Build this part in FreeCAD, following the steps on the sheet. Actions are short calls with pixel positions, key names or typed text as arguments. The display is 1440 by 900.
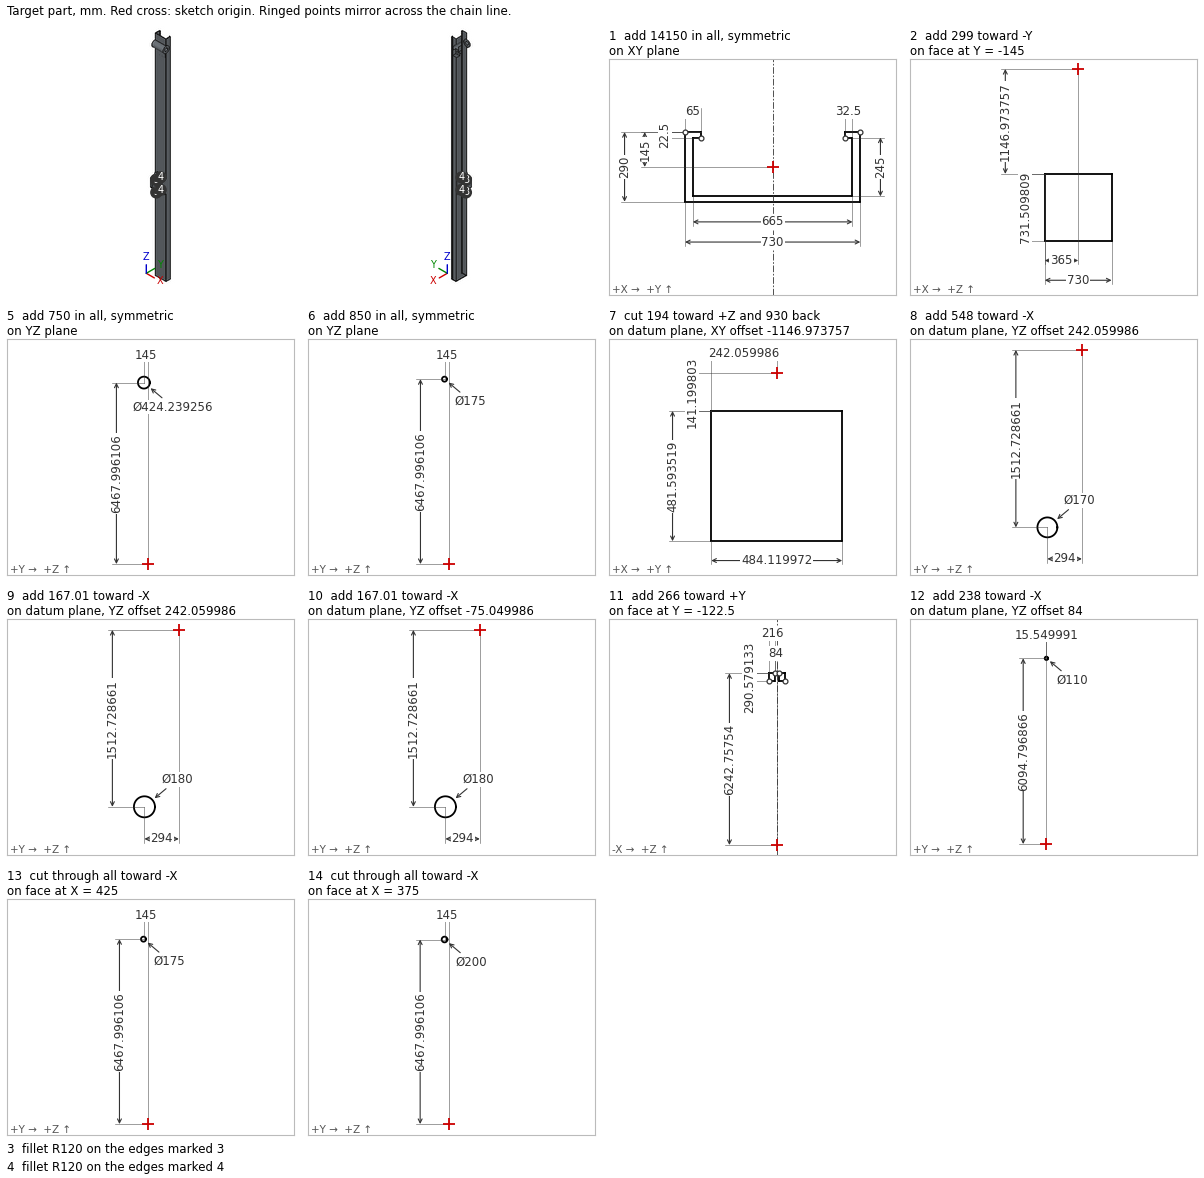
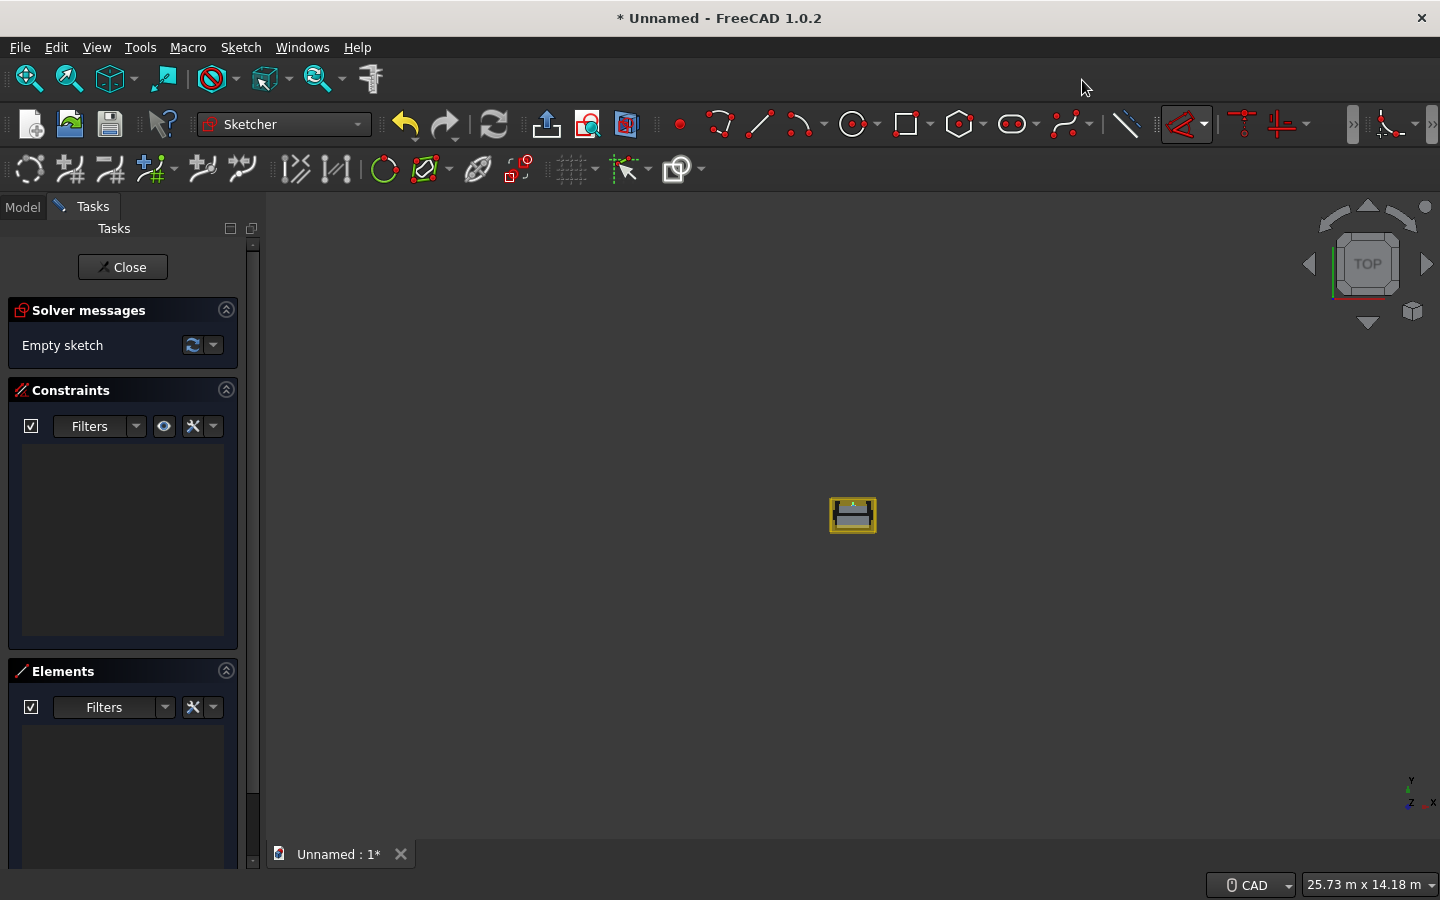
click(628, 124)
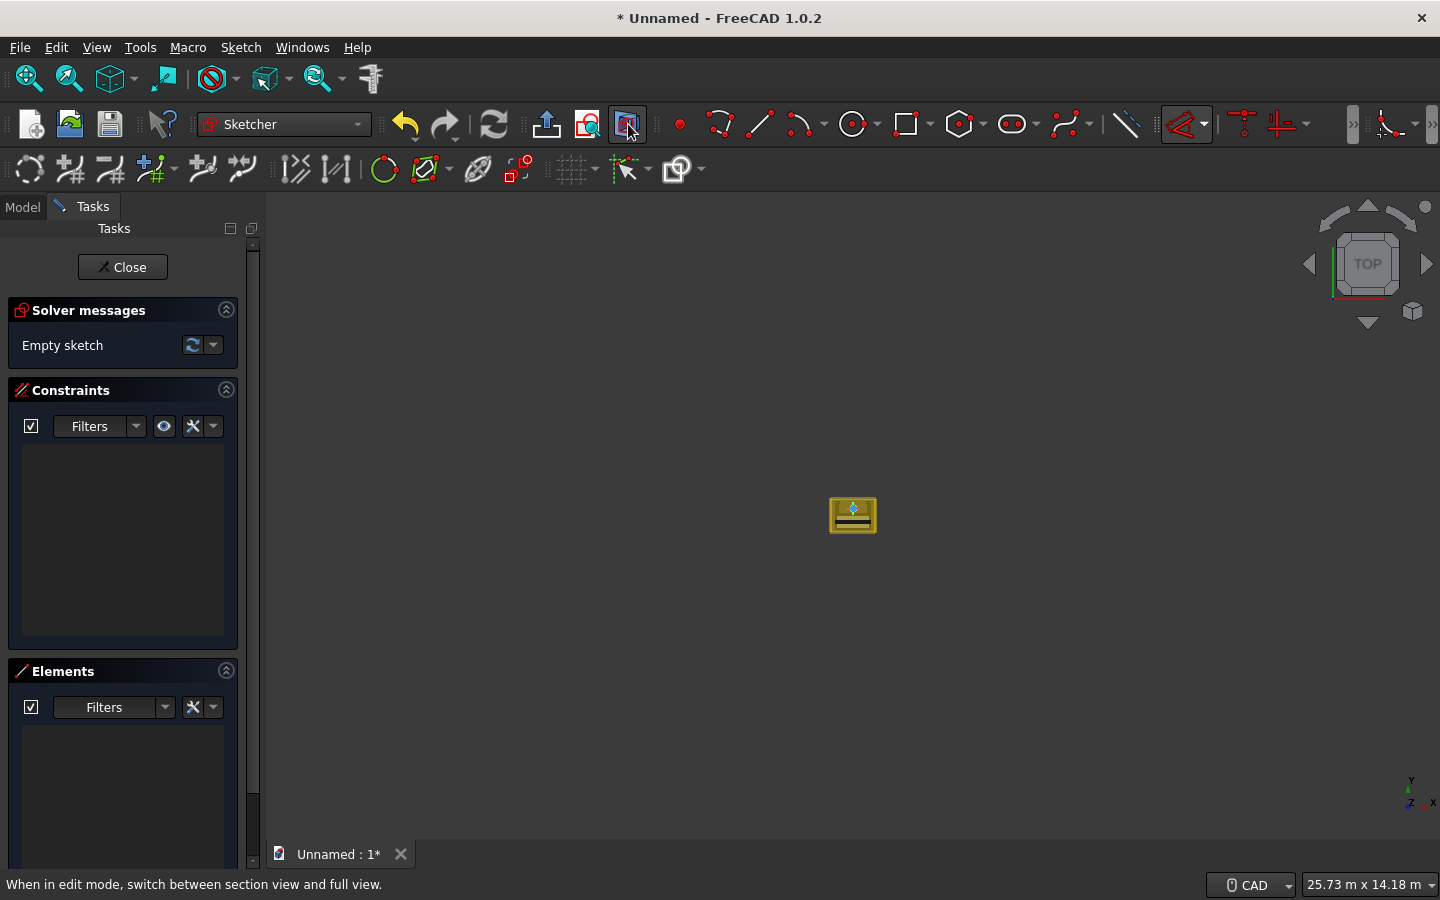
scroll(858, 523, up, 13)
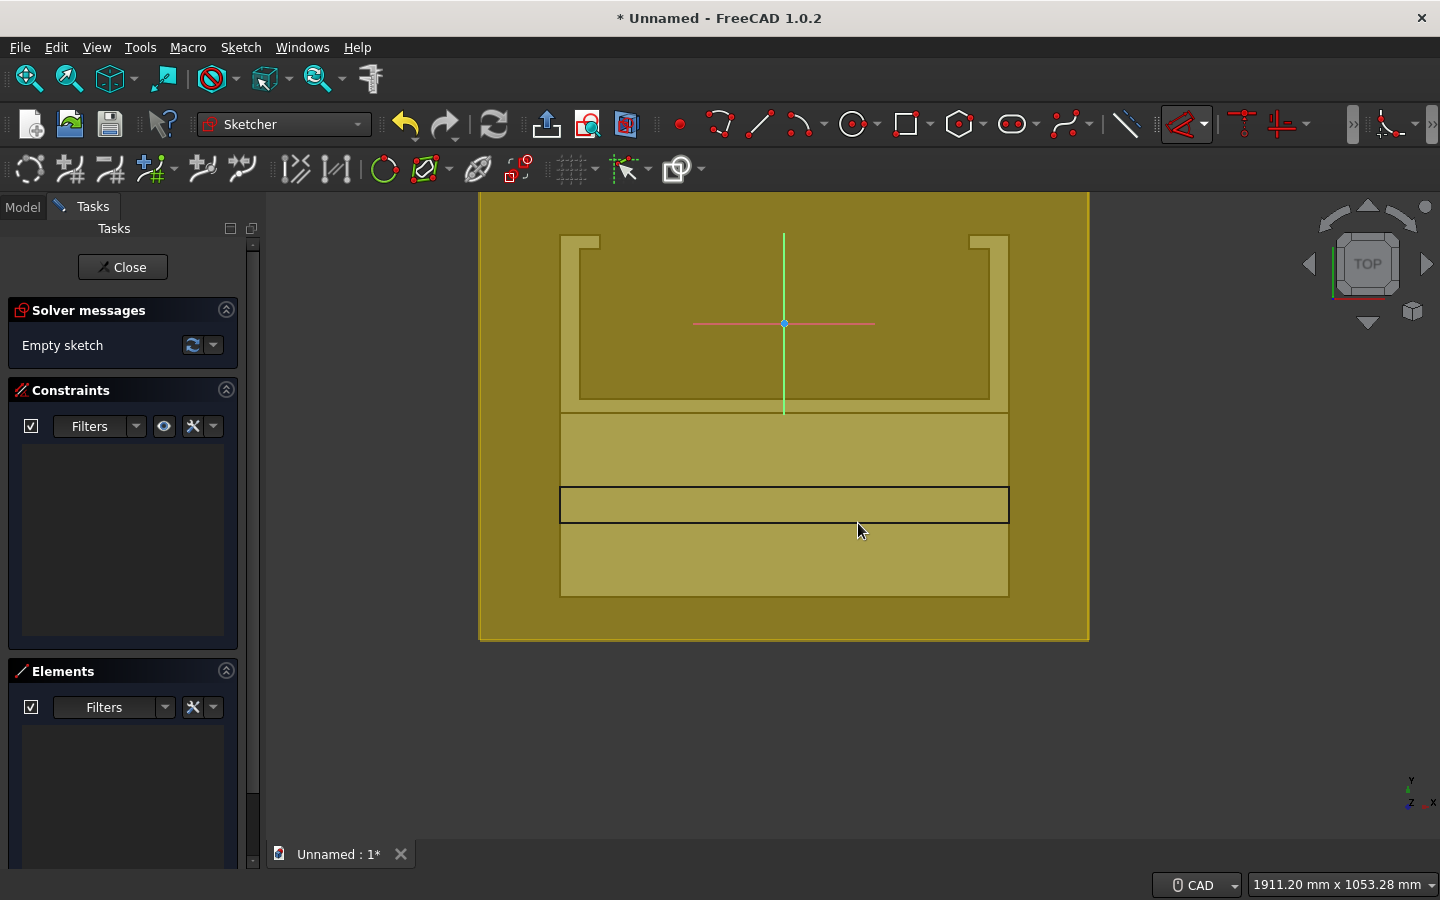
key(g)
key(r)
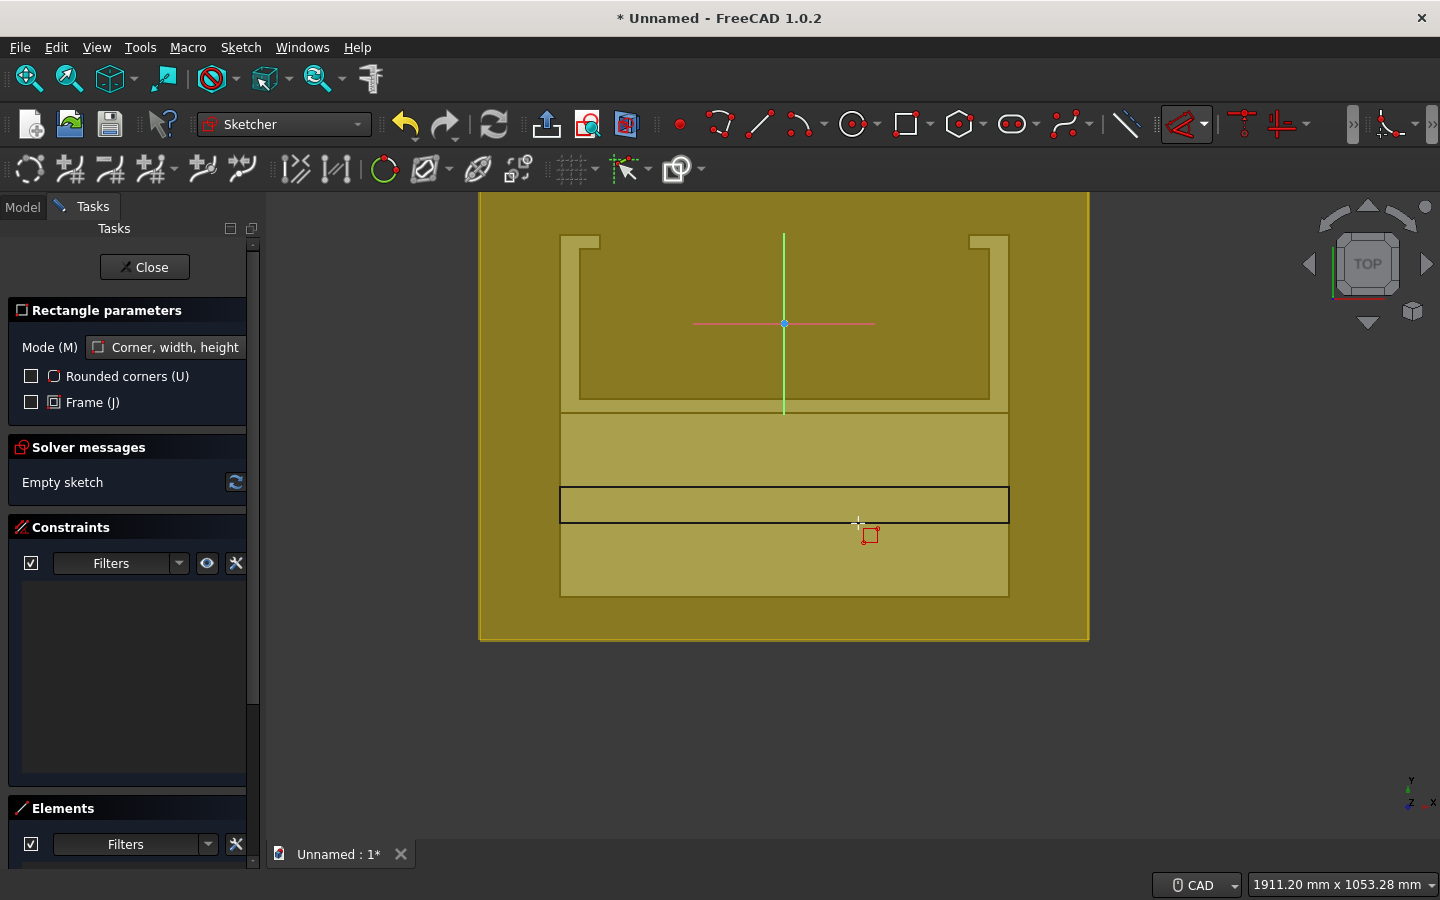
click(636, 411)
click(933, 706)
key(Escape)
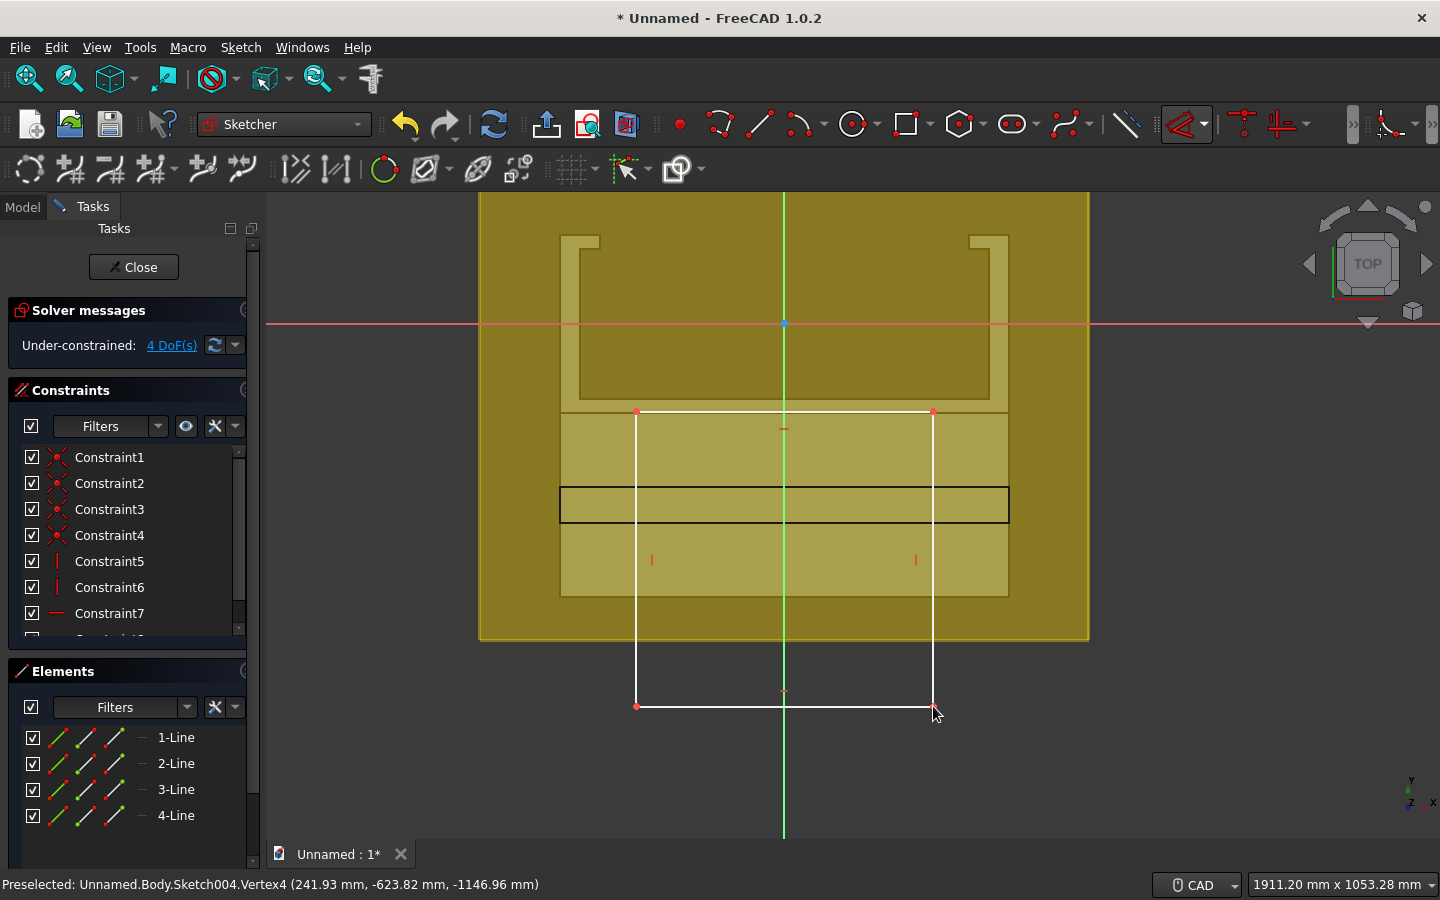
click(636, 500)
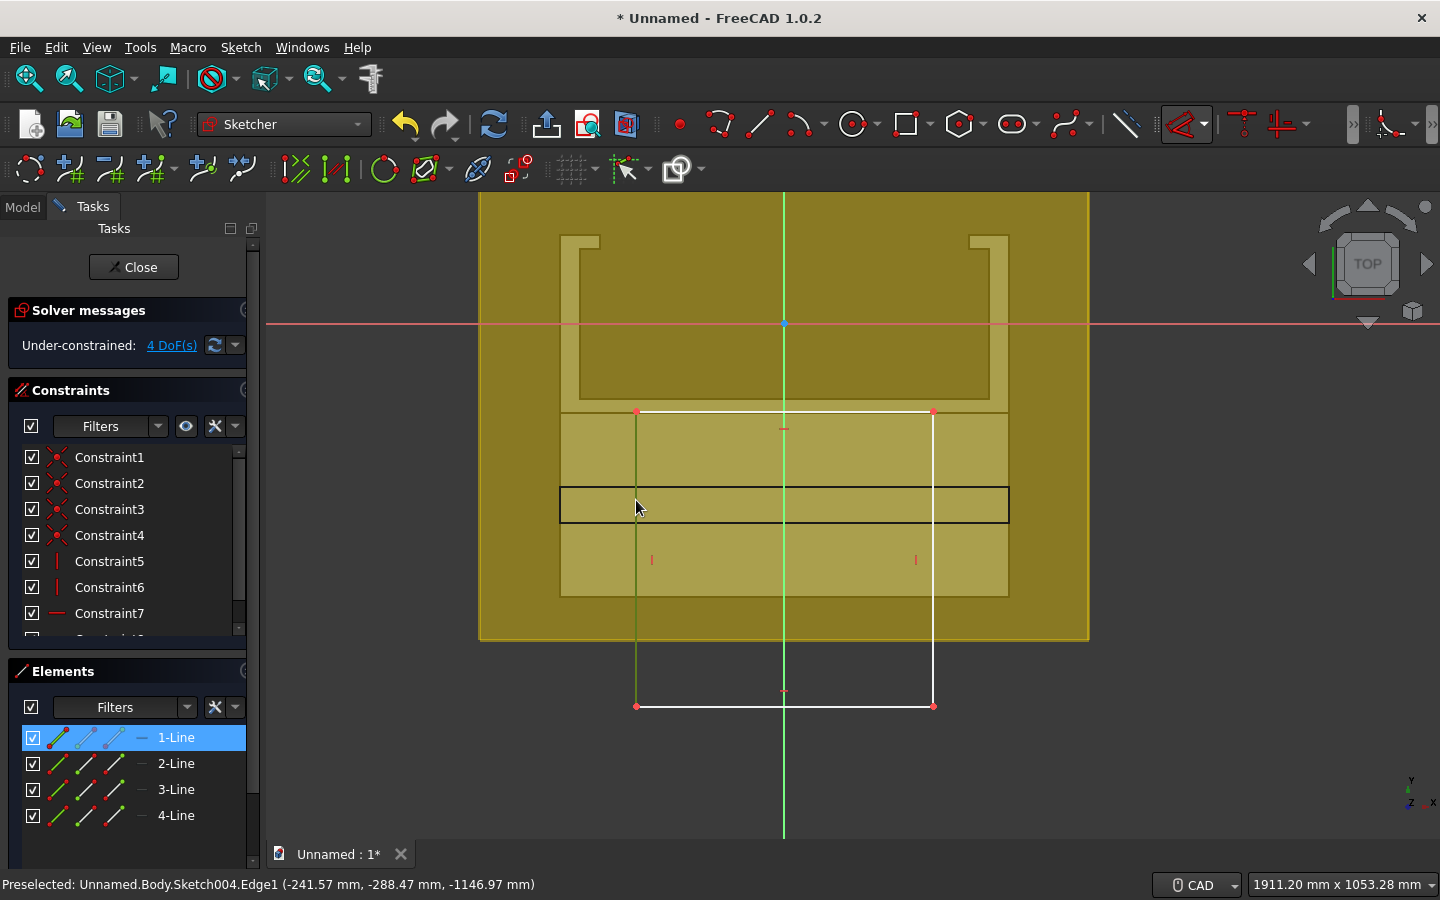
click(1206, 124)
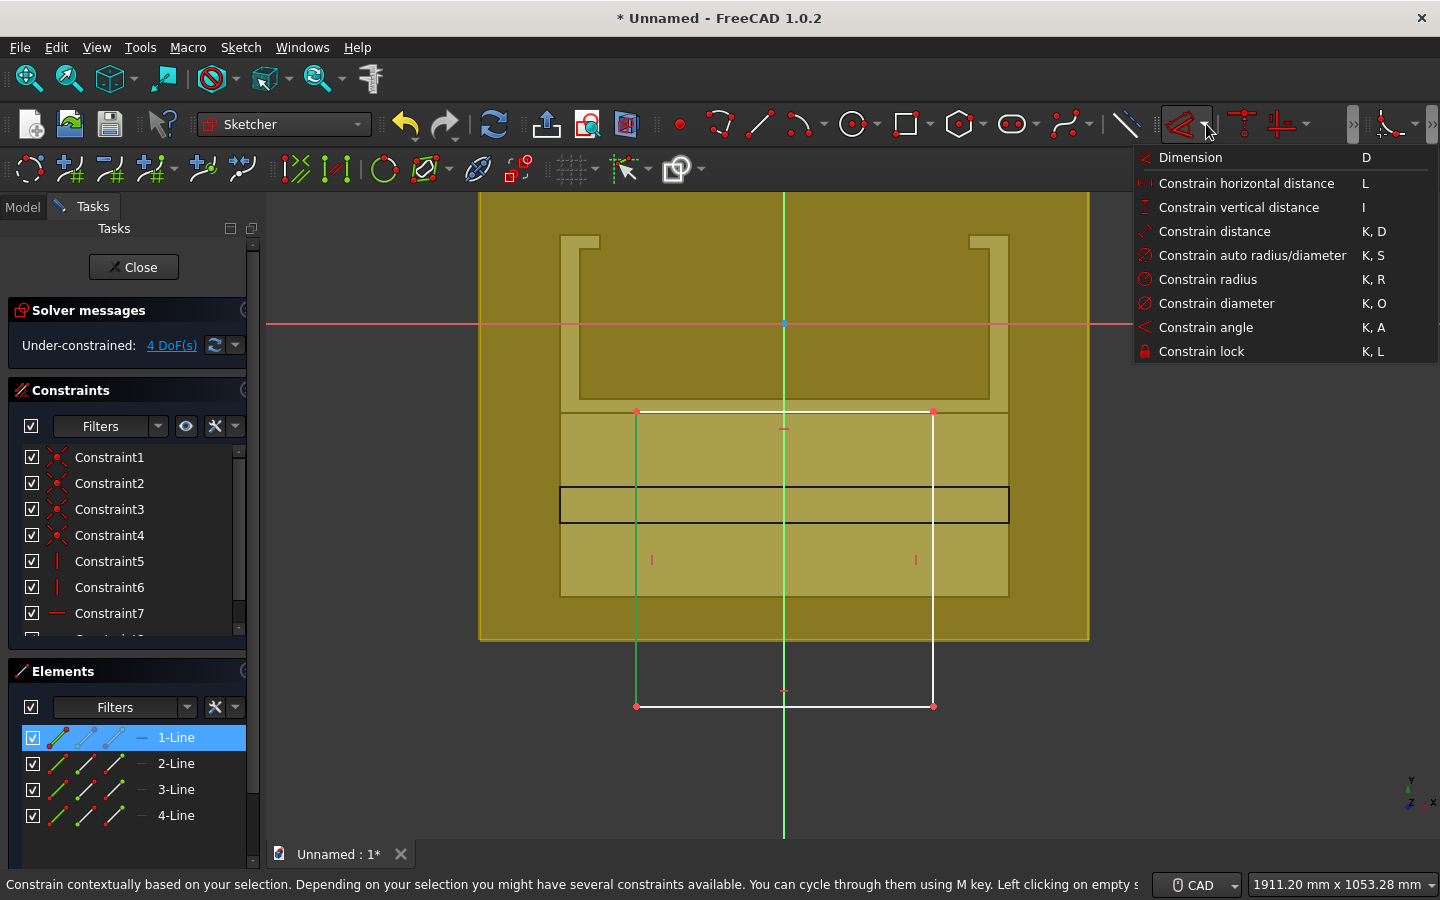
click(1286, 207)